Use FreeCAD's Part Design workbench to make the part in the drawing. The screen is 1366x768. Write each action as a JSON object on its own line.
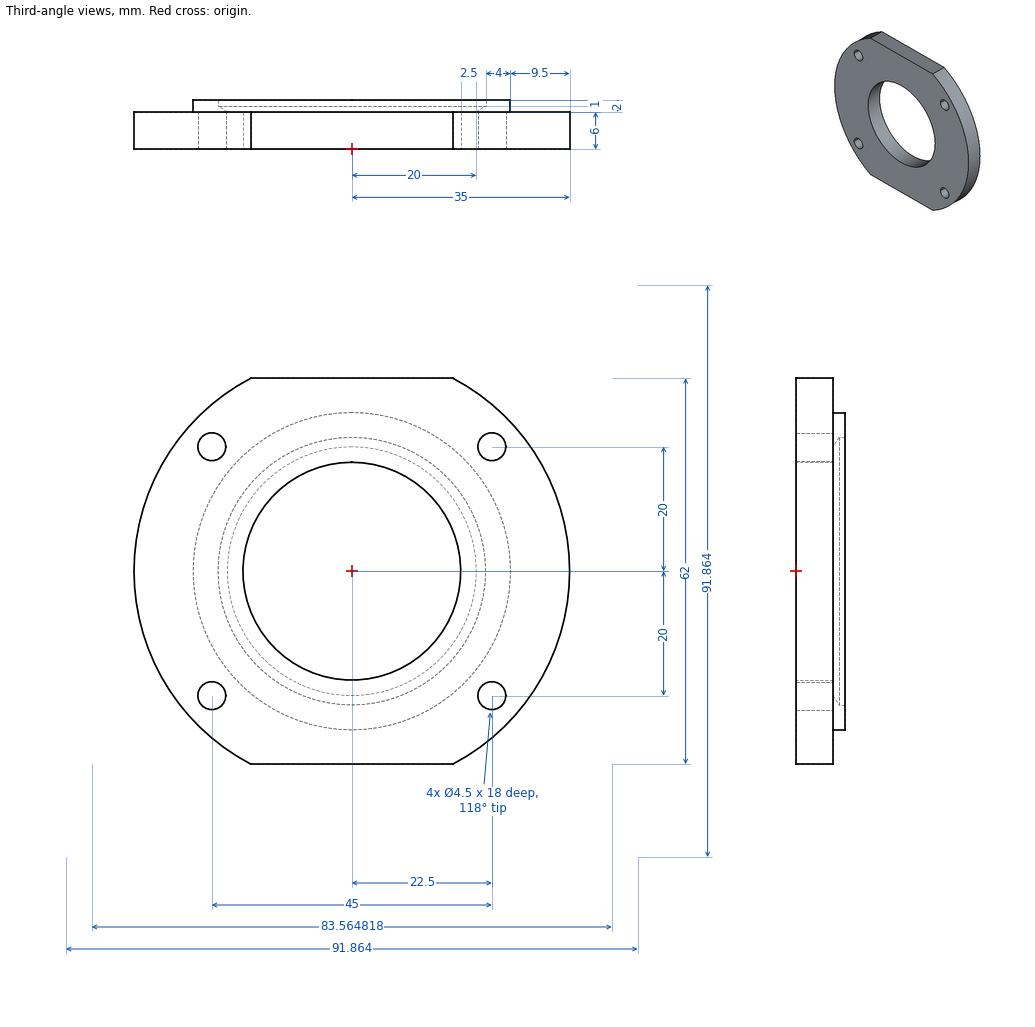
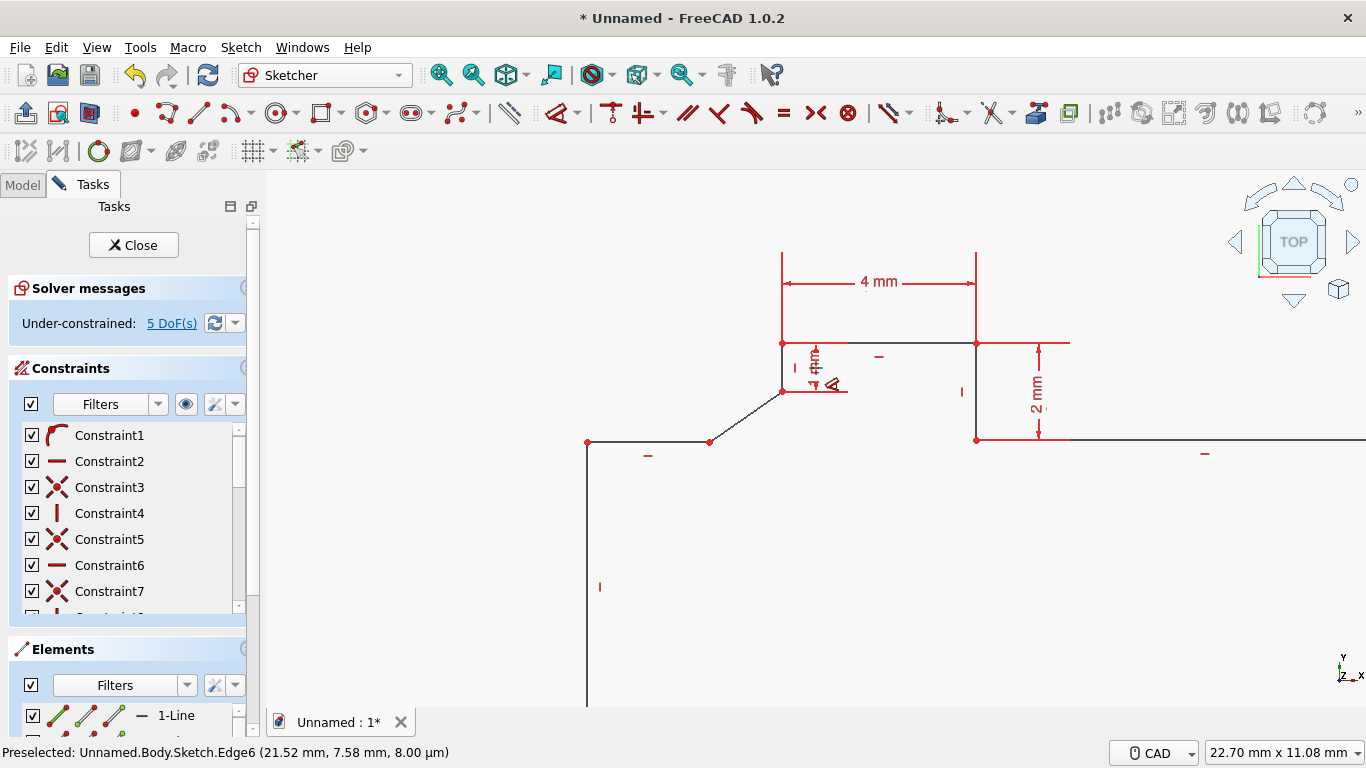
{"action": "left_click", "coordinate": [587, 529]}
{"action": "left_click", "coordinate": [553, 561]}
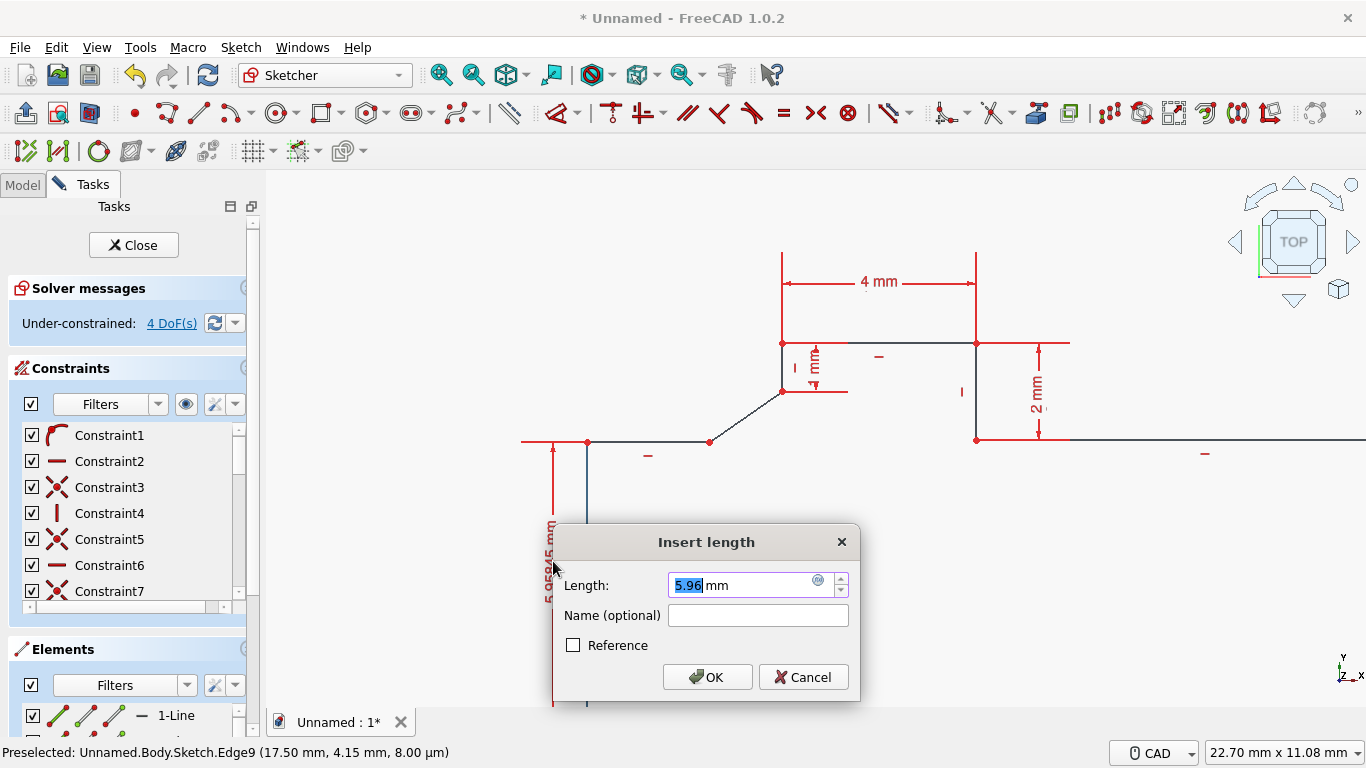
{"action": "type", "text": "6"}
{"action": "key", "text": "Return"}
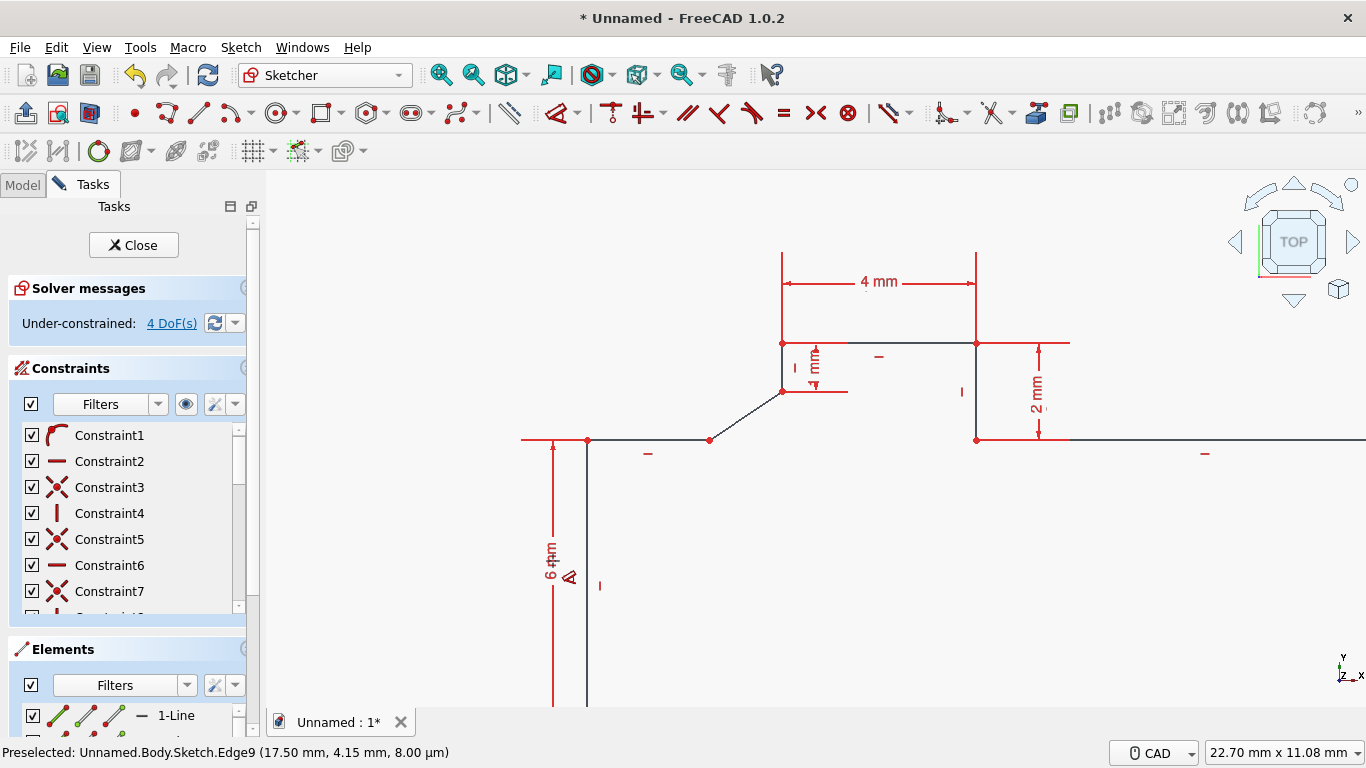
{"action": "left_click", "coordinate": [1114, 440]}
{"action": "left_click", "coordinate": [1140, 406]}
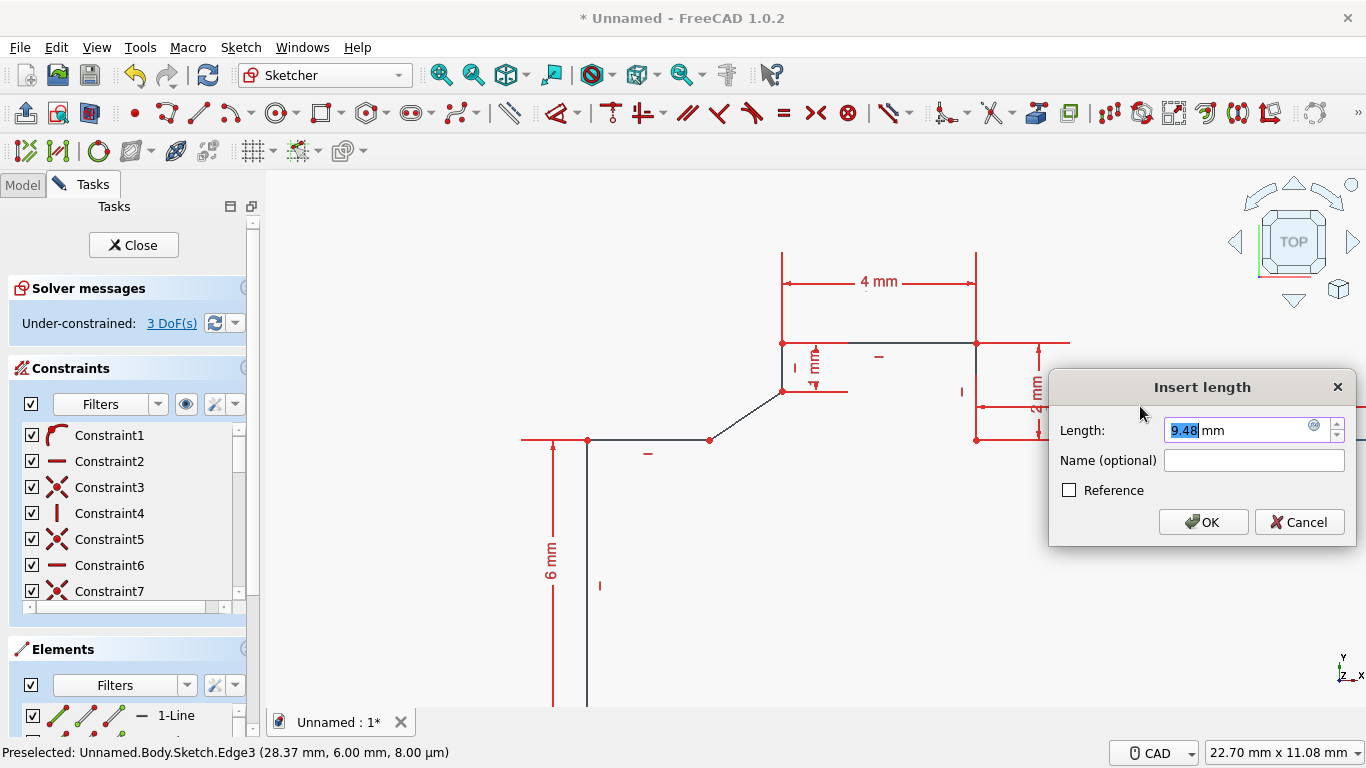
{"action": "type", "text": "9.5"}
{"action": "key", "text": "Return"}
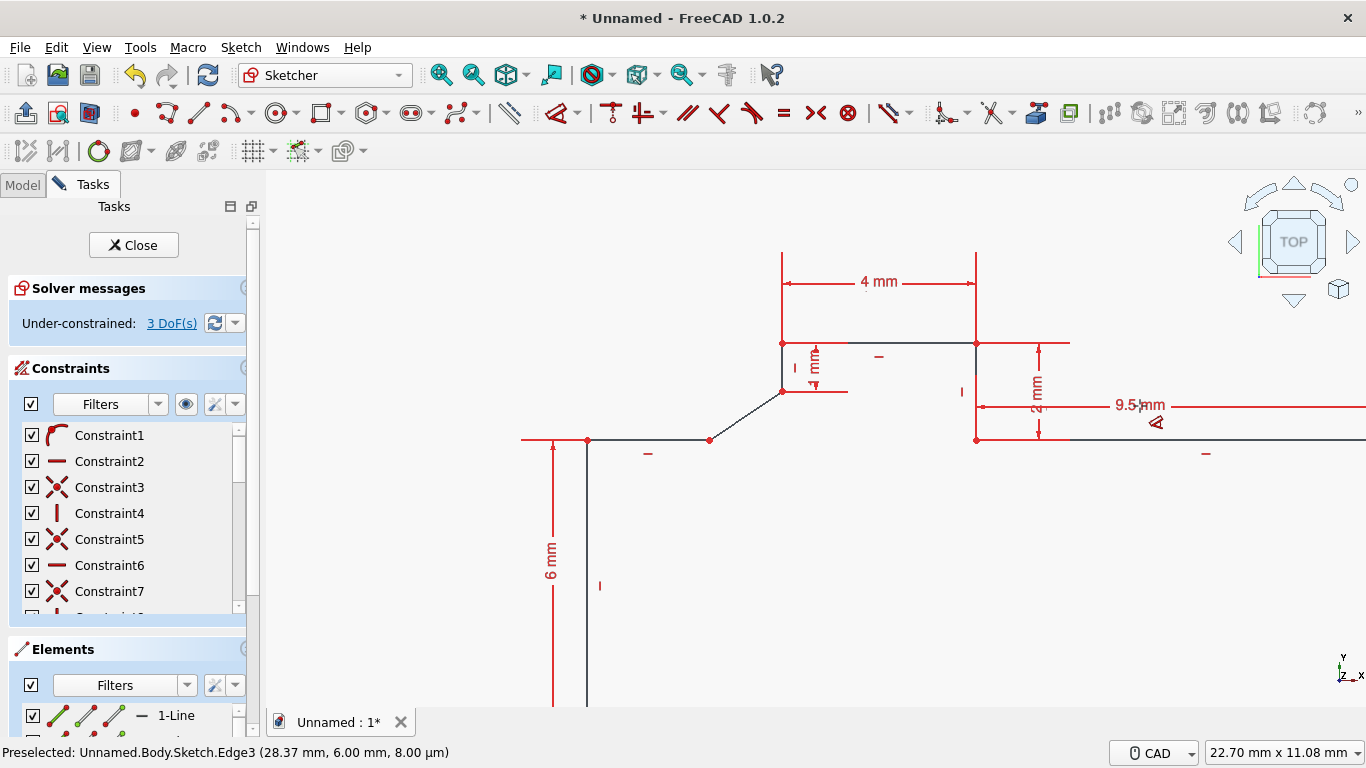
{"action": "left_click", "coordinate": [673, 440]}
{"action": "left_click", "coordinate": [649, 406]}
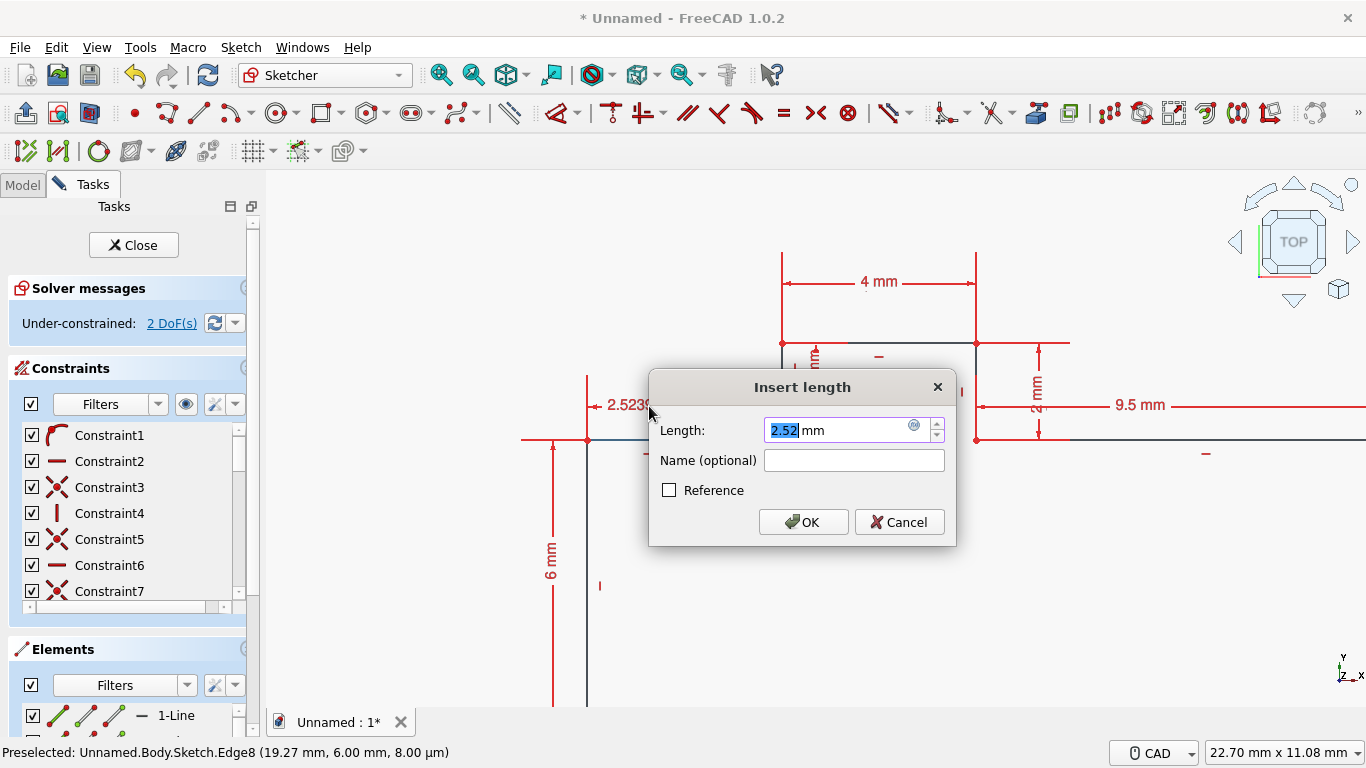
{"action": "type", "text": "2.5"}
{"action": "key", "text": "Return"}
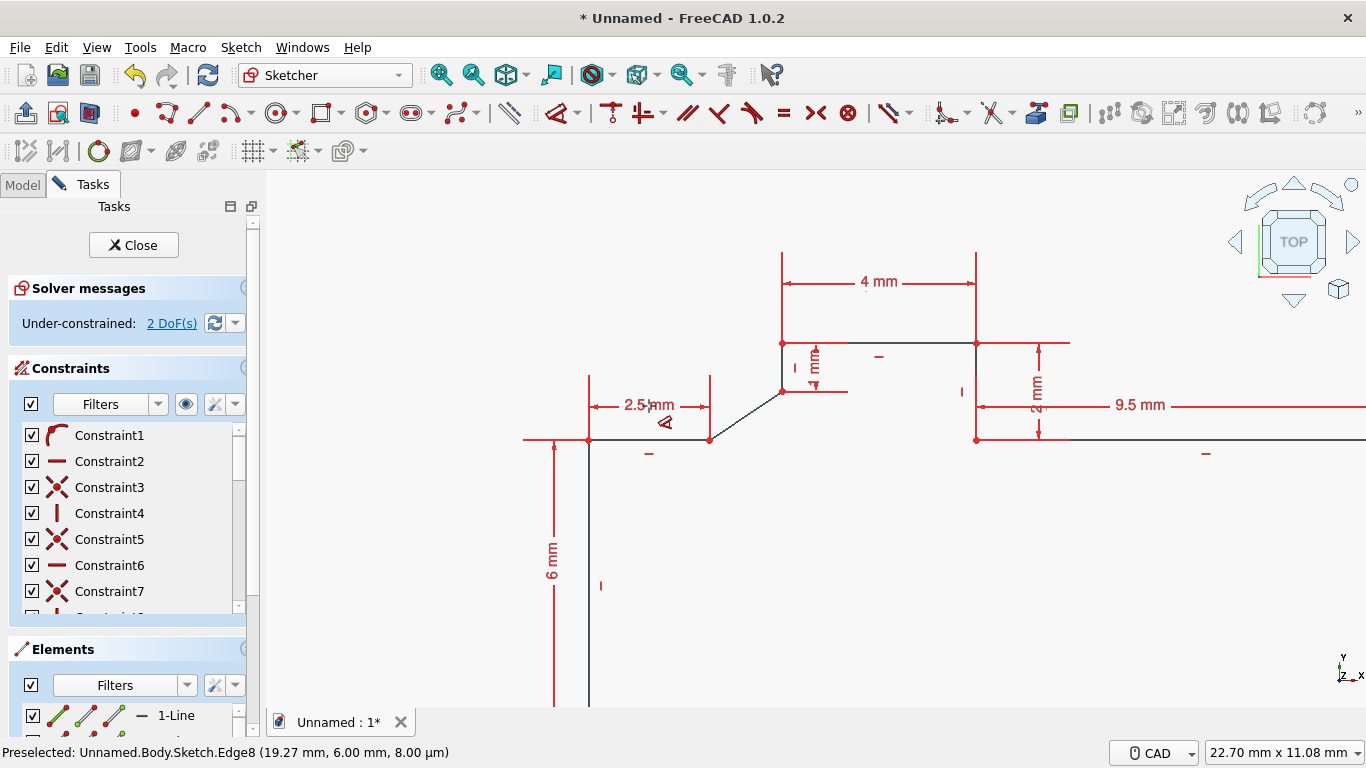
{"action": "scroll", "coordinate": [841, 381], "scroll_direction": "down", "scroll_amount": 5}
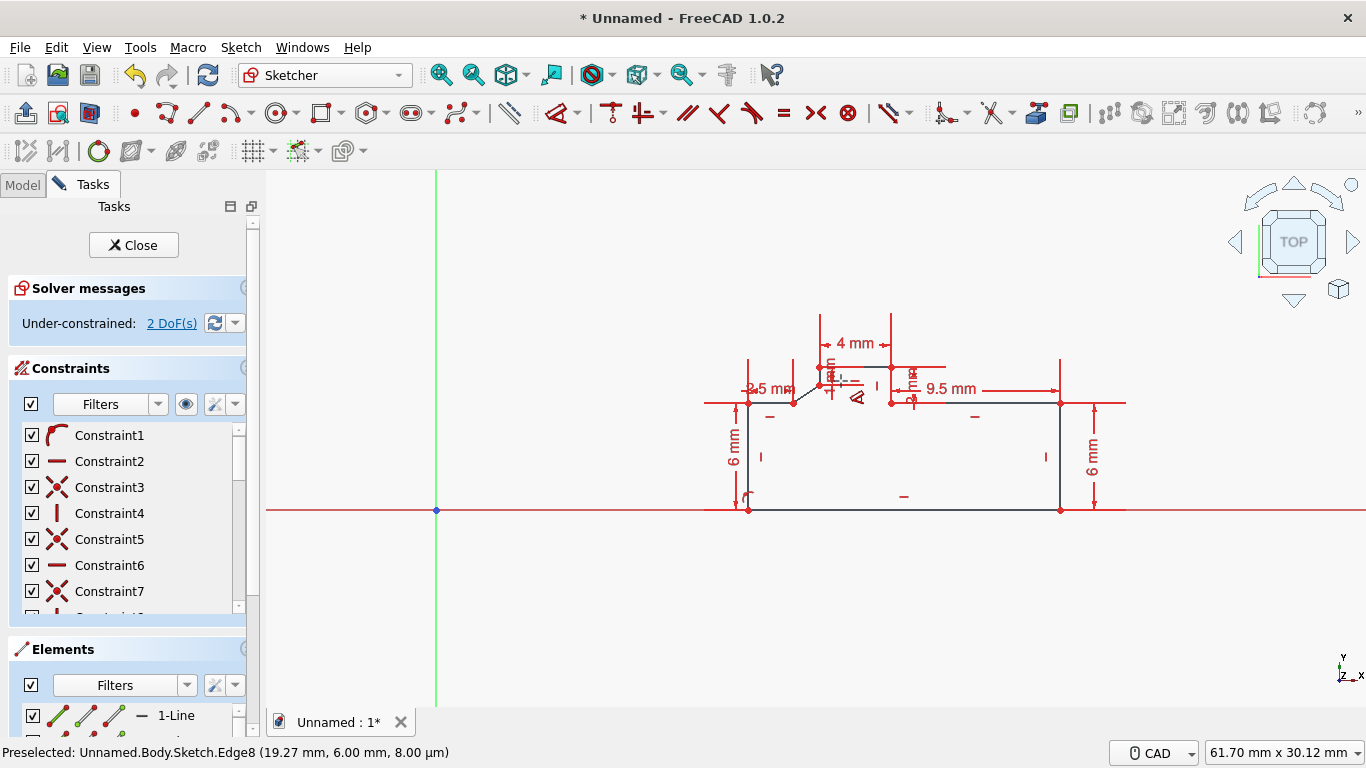
{"action": "left_click", "coordinate": [1060, 510]}
{"action": "left_click", "coordinate": [748, 544]}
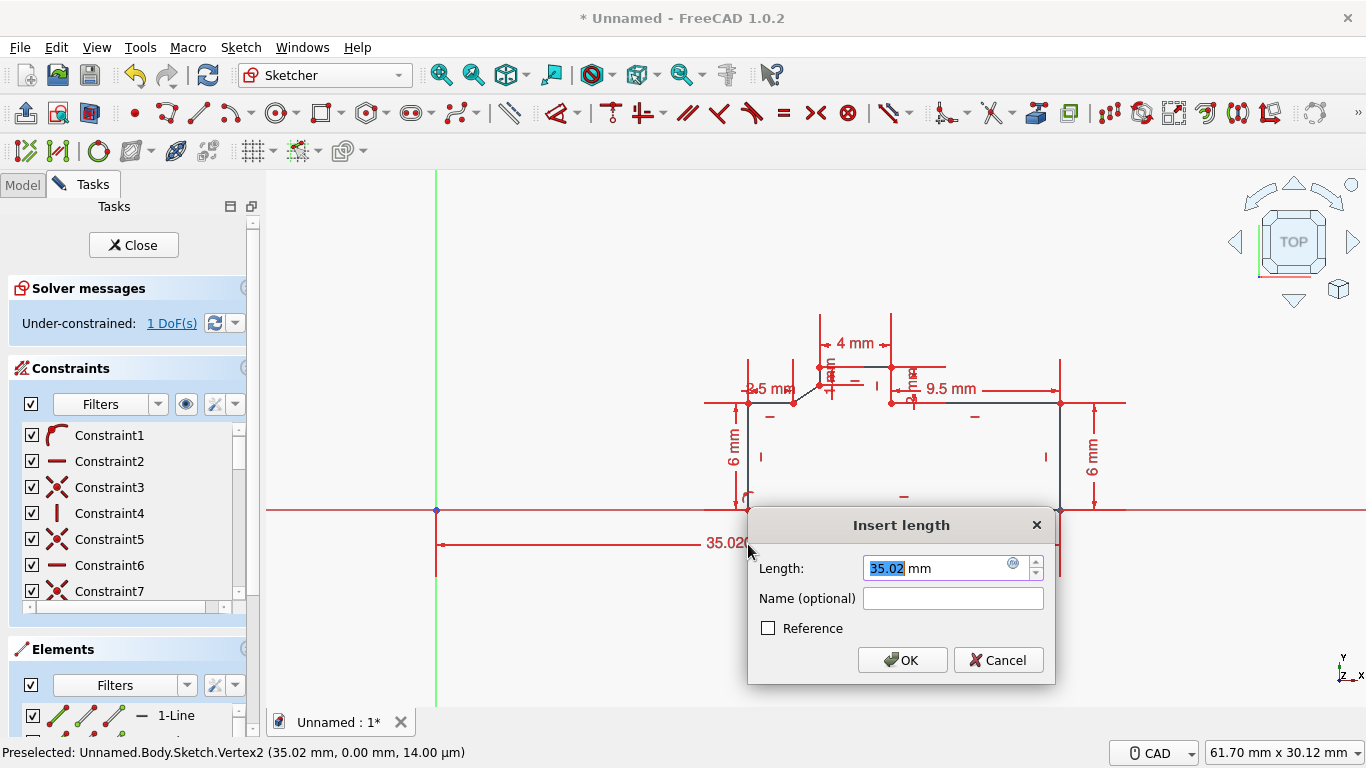
{"action": "type", "text": "35"}
{"action": "key", "text": "Return"}